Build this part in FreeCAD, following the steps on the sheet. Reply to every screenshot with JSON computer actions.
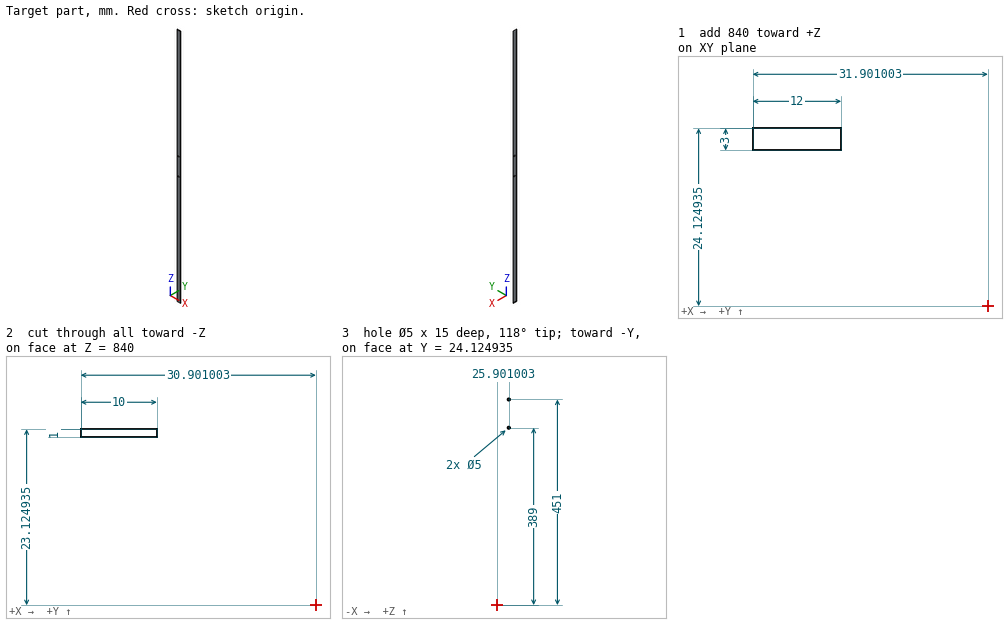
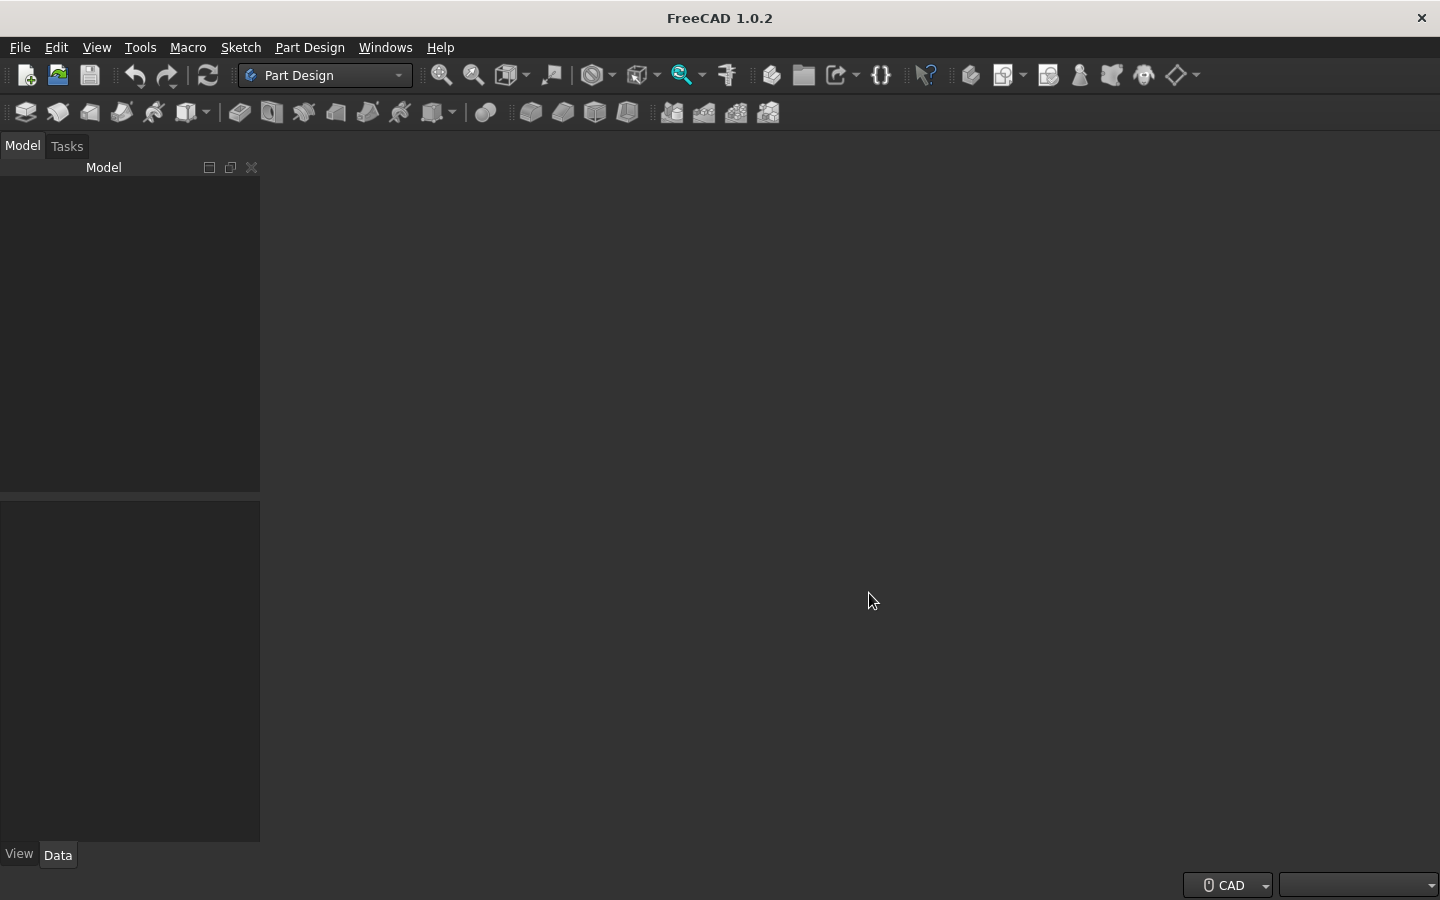
{"action": "left_click", "coordinate": [26, 76]}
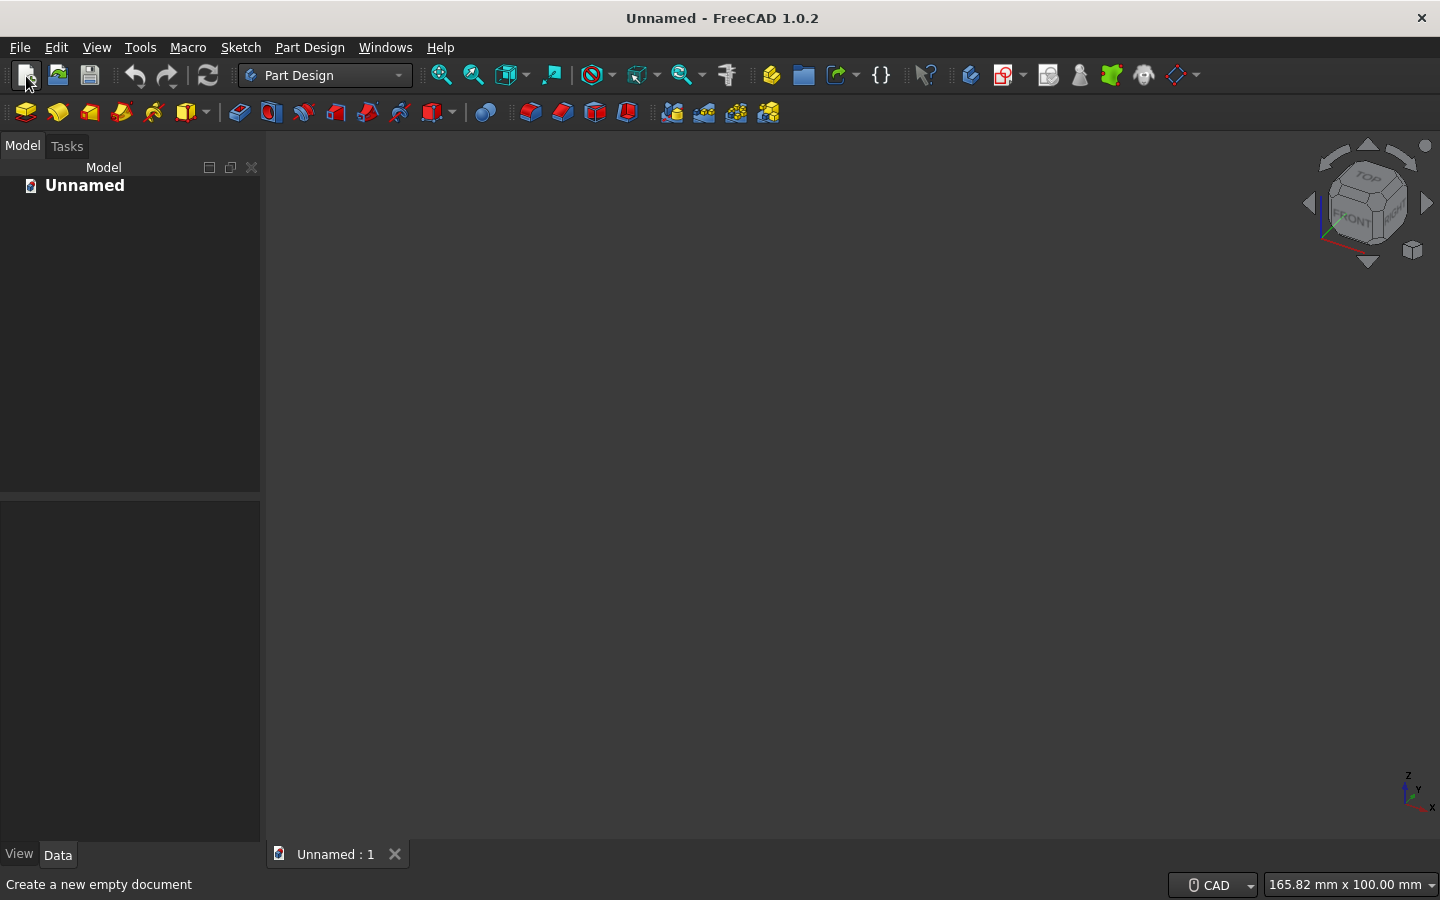
{"action": "left_click", "coordinate": [1004, 76]}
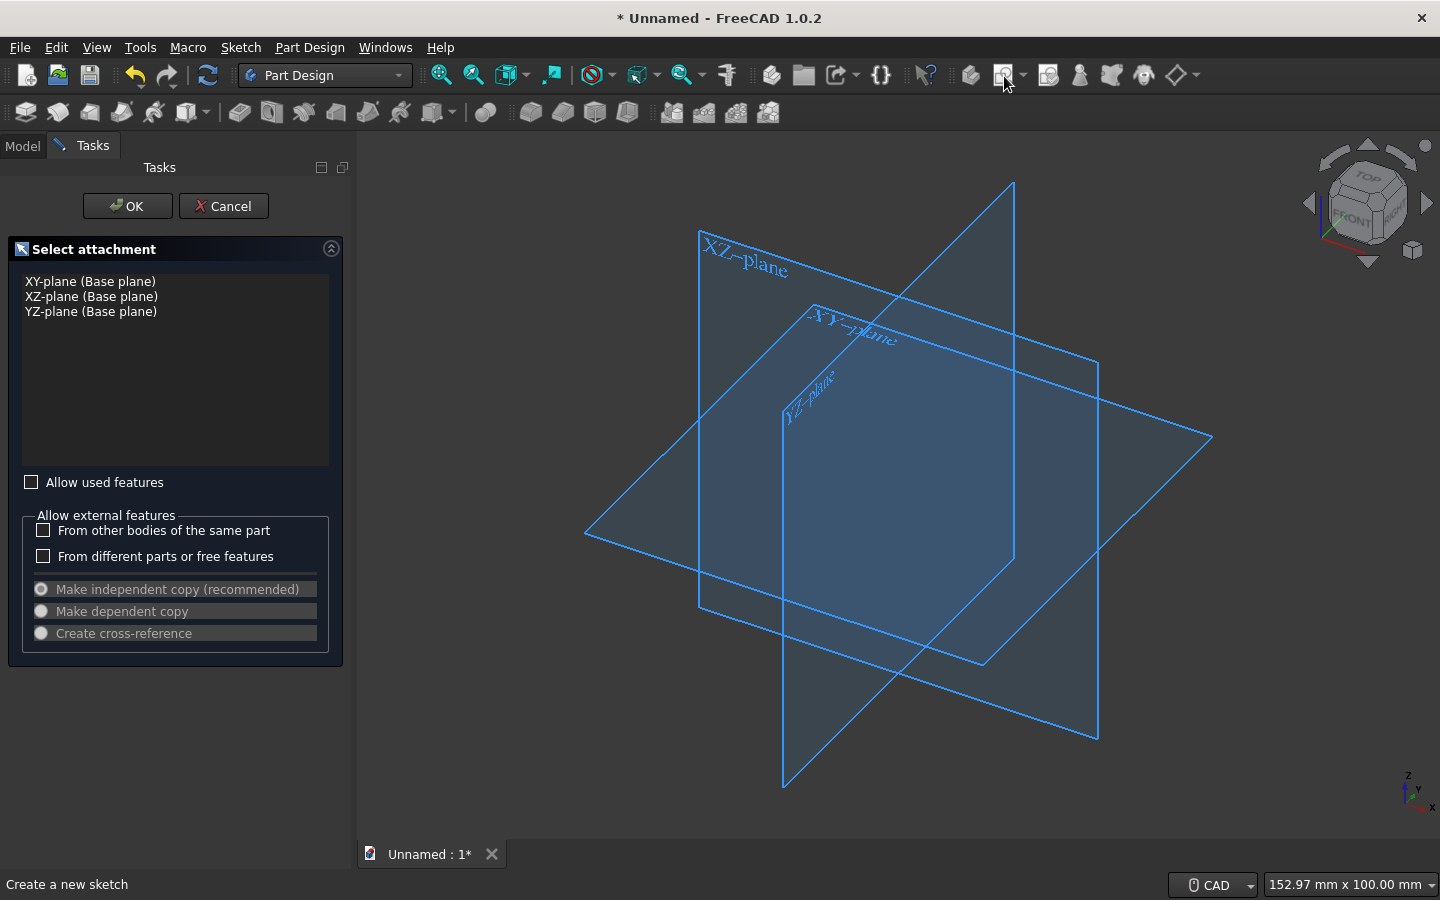
{"action": "left_click", "coordinate": [82, 282]}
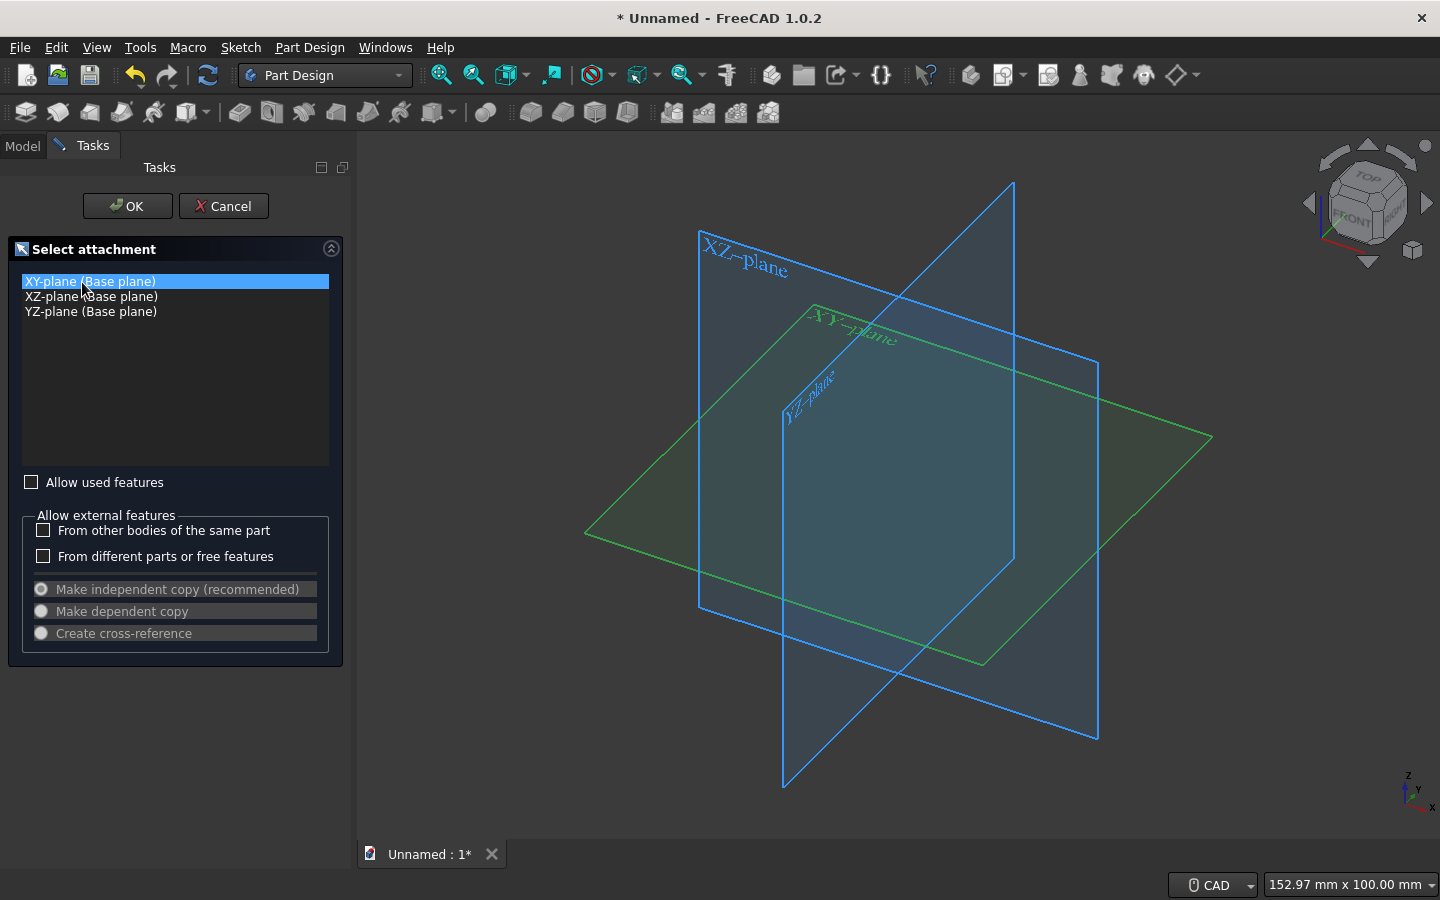
{"action": "left_click", "coordinate": [128, 206]}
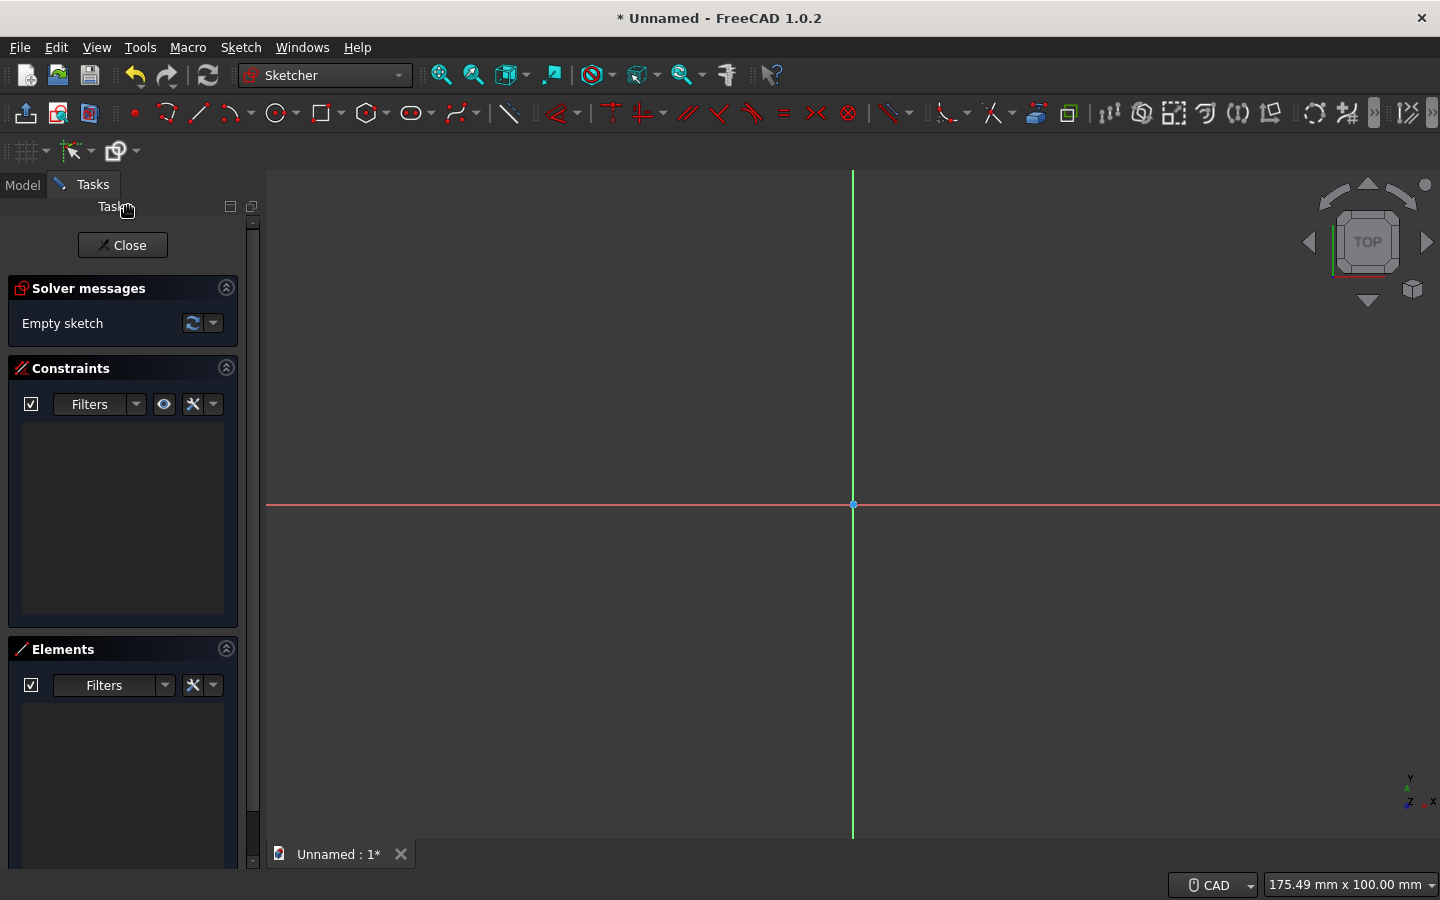
{"action": "scroll", "coordinate": [667, 334], "scroll_direction": "up", "scroll_amount": 11}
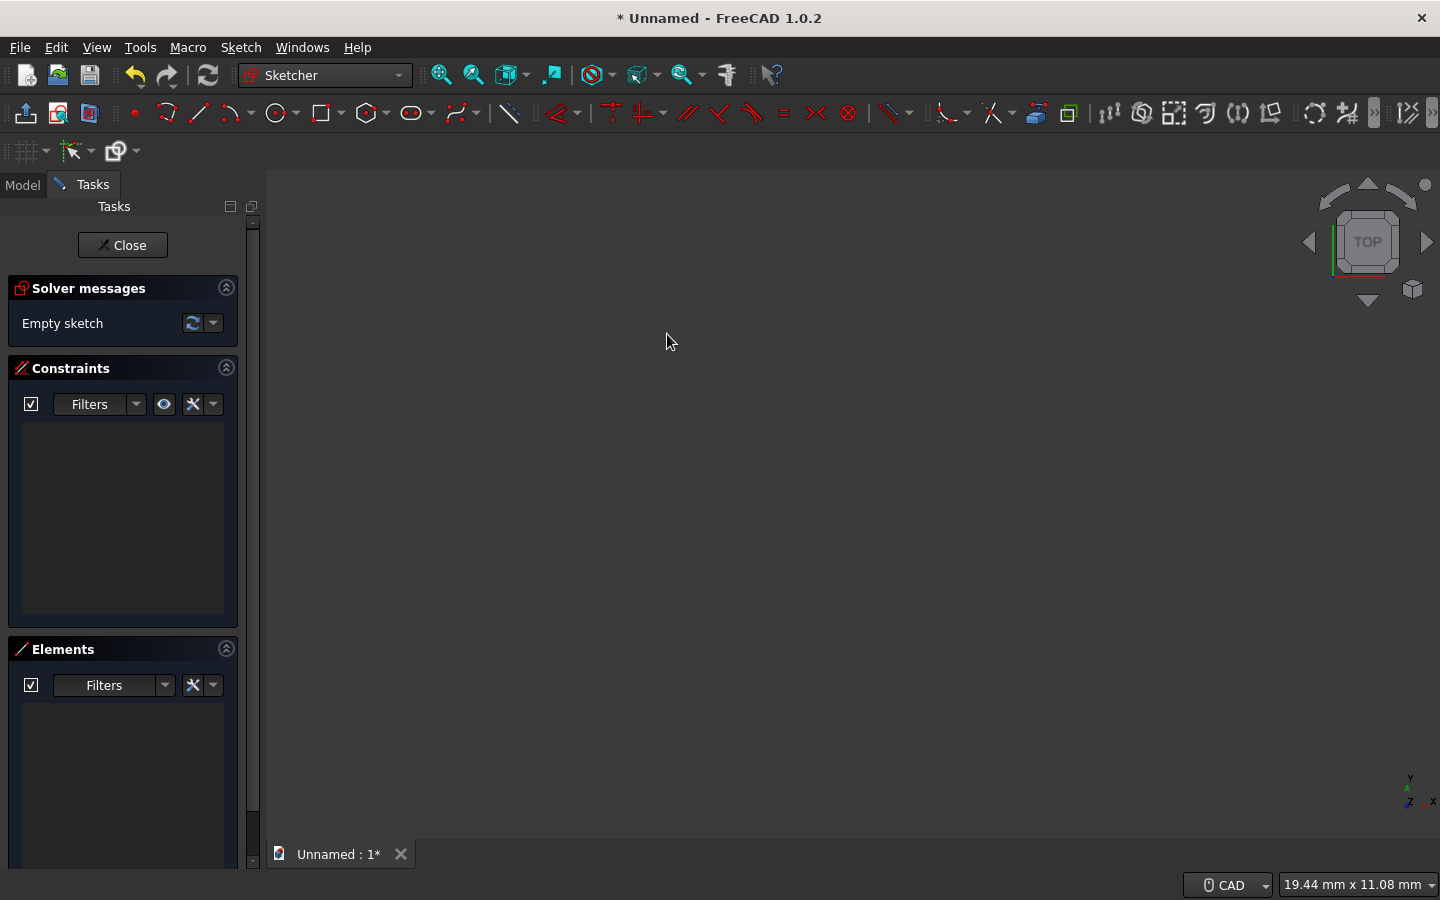
{"action": "left_click", "coordinate": [322, 114]}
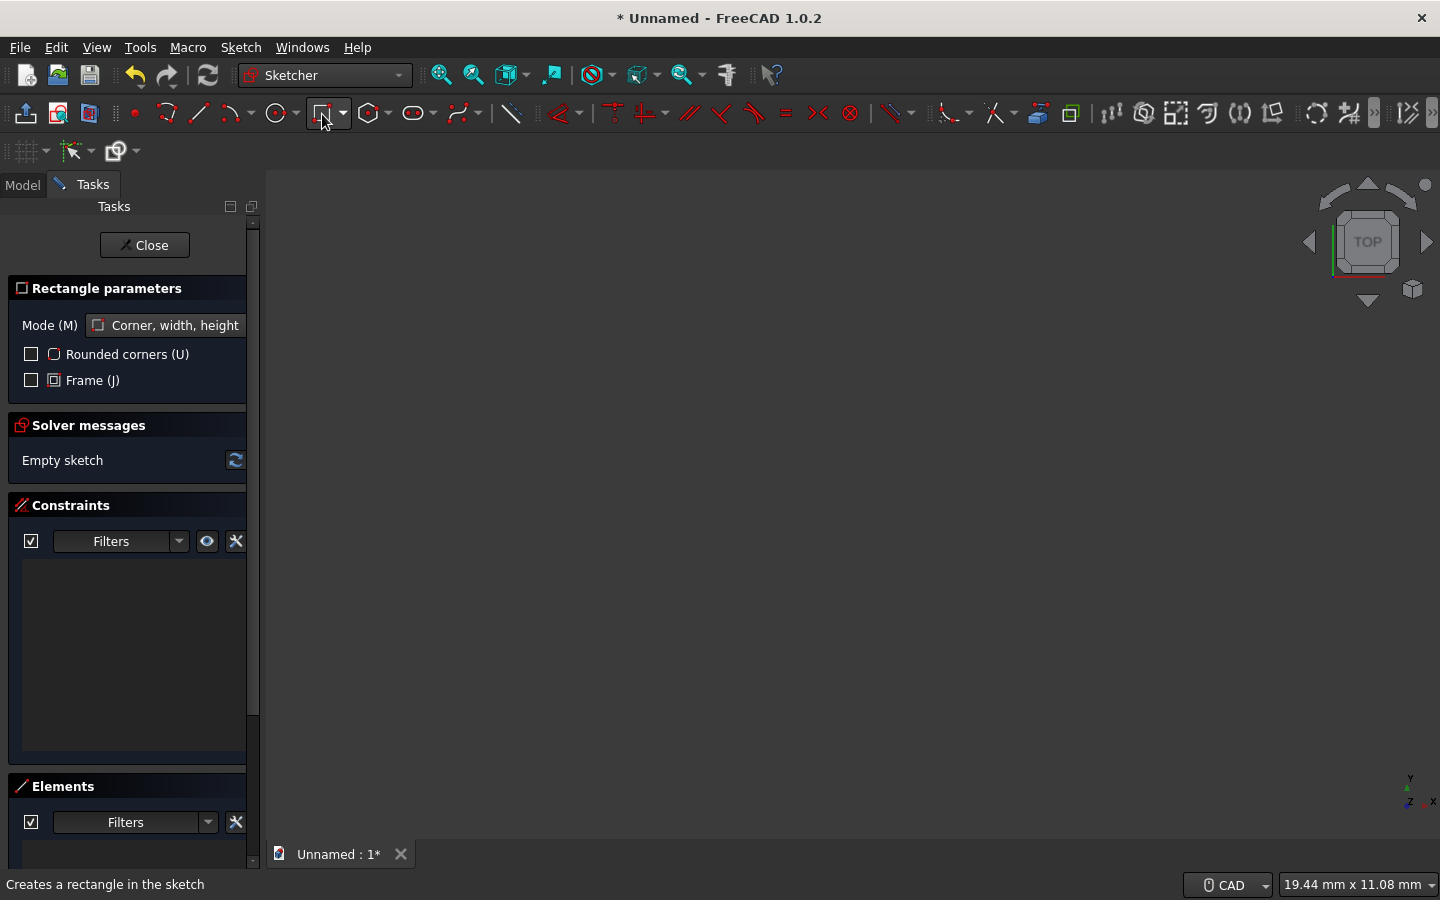
{"action": "left_click", "coordinate": [417, 414]}
{"action": "mouse_move", "coordinate": [1141, 595]}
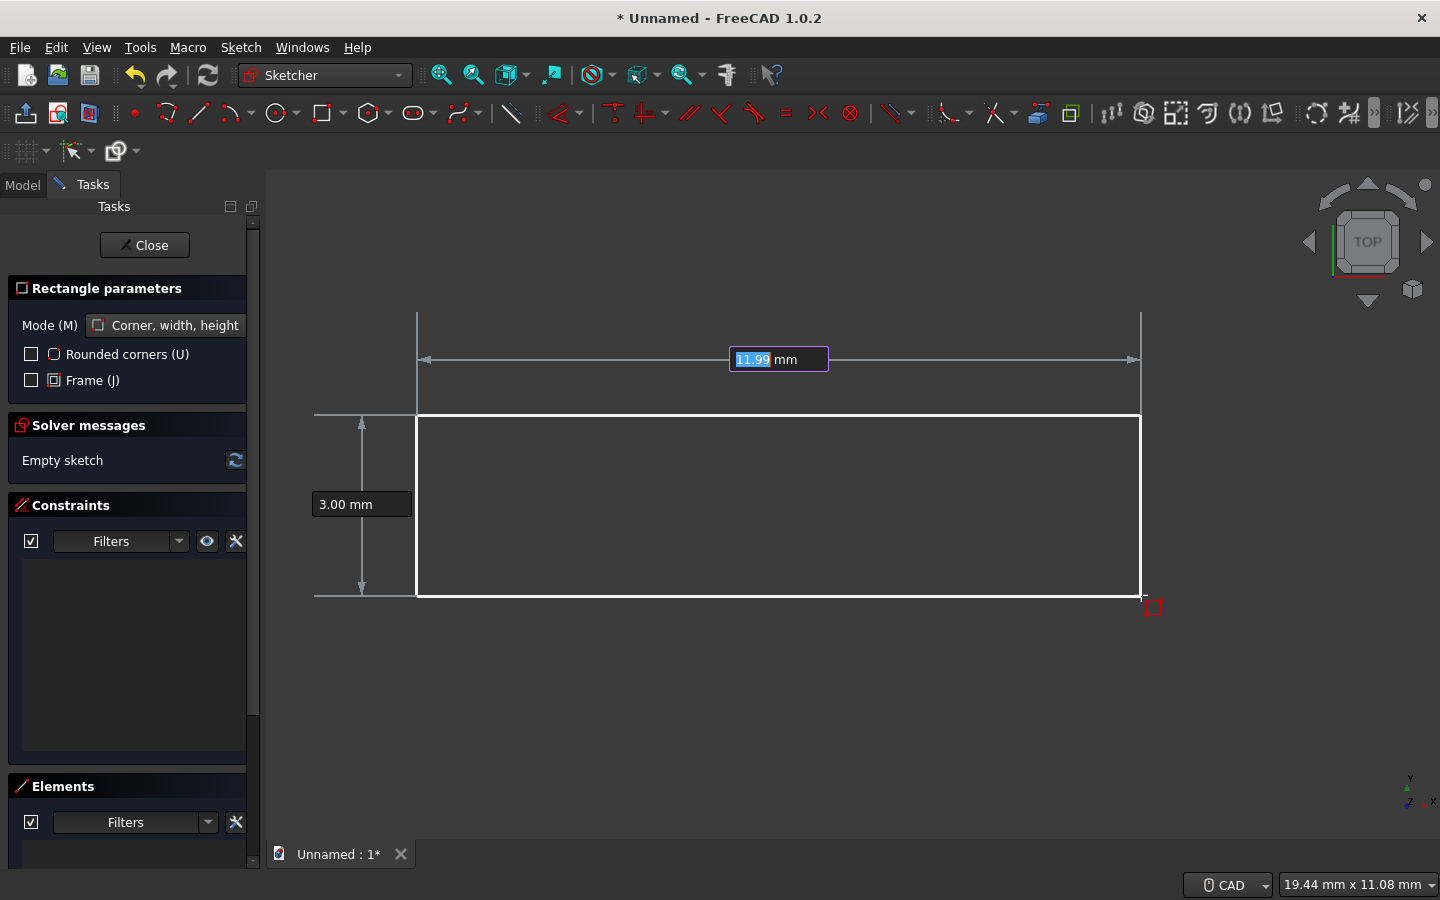
{"action": "type", "text": "12"}
{"action": "key", "text": "Tab"}
{"action": "type", "text": "3"}
{"action": "key", "text": "Return"}
{"action": "key", "text": "Escape"}